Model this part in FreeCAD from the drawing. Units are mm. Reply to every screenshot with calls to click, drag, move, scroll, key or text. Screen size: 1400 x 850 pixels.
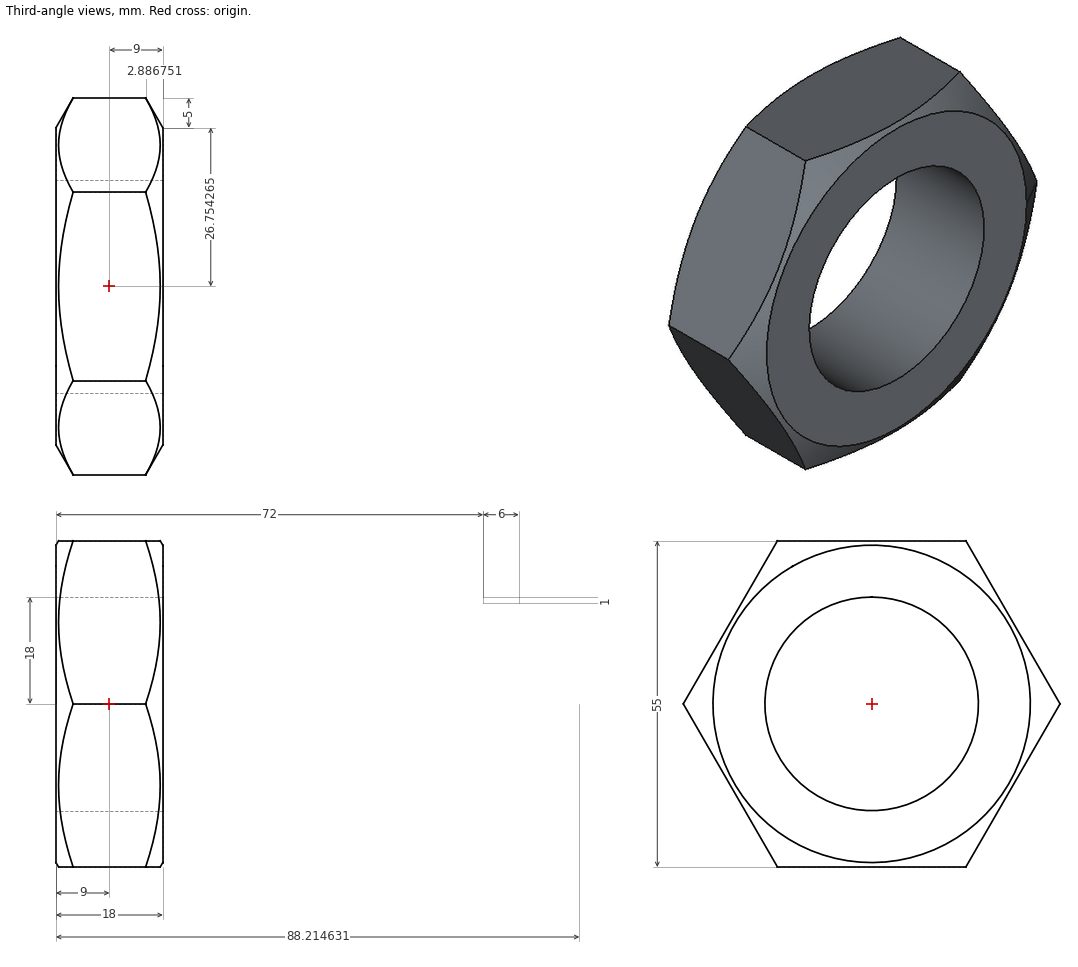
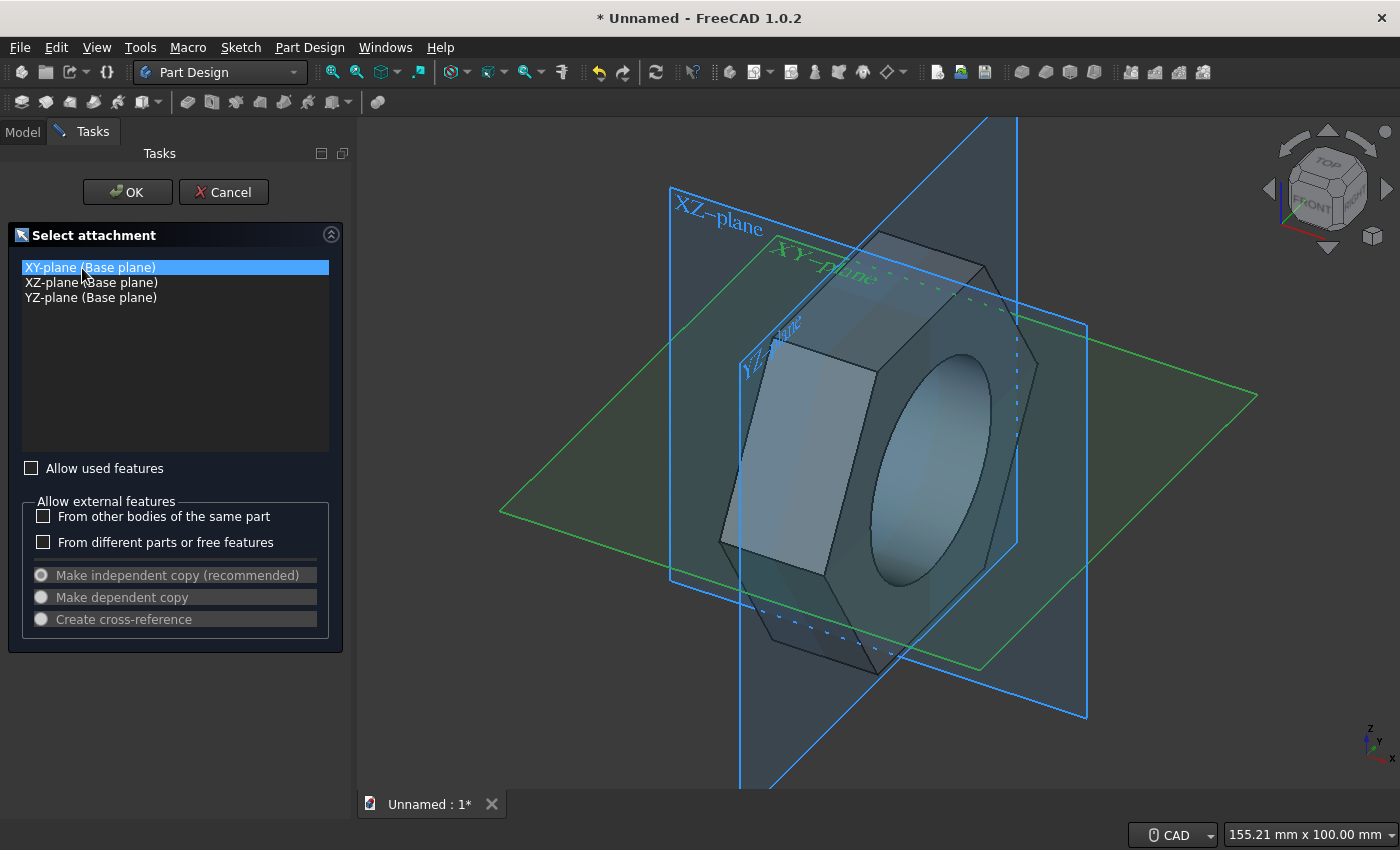
click(128, 192)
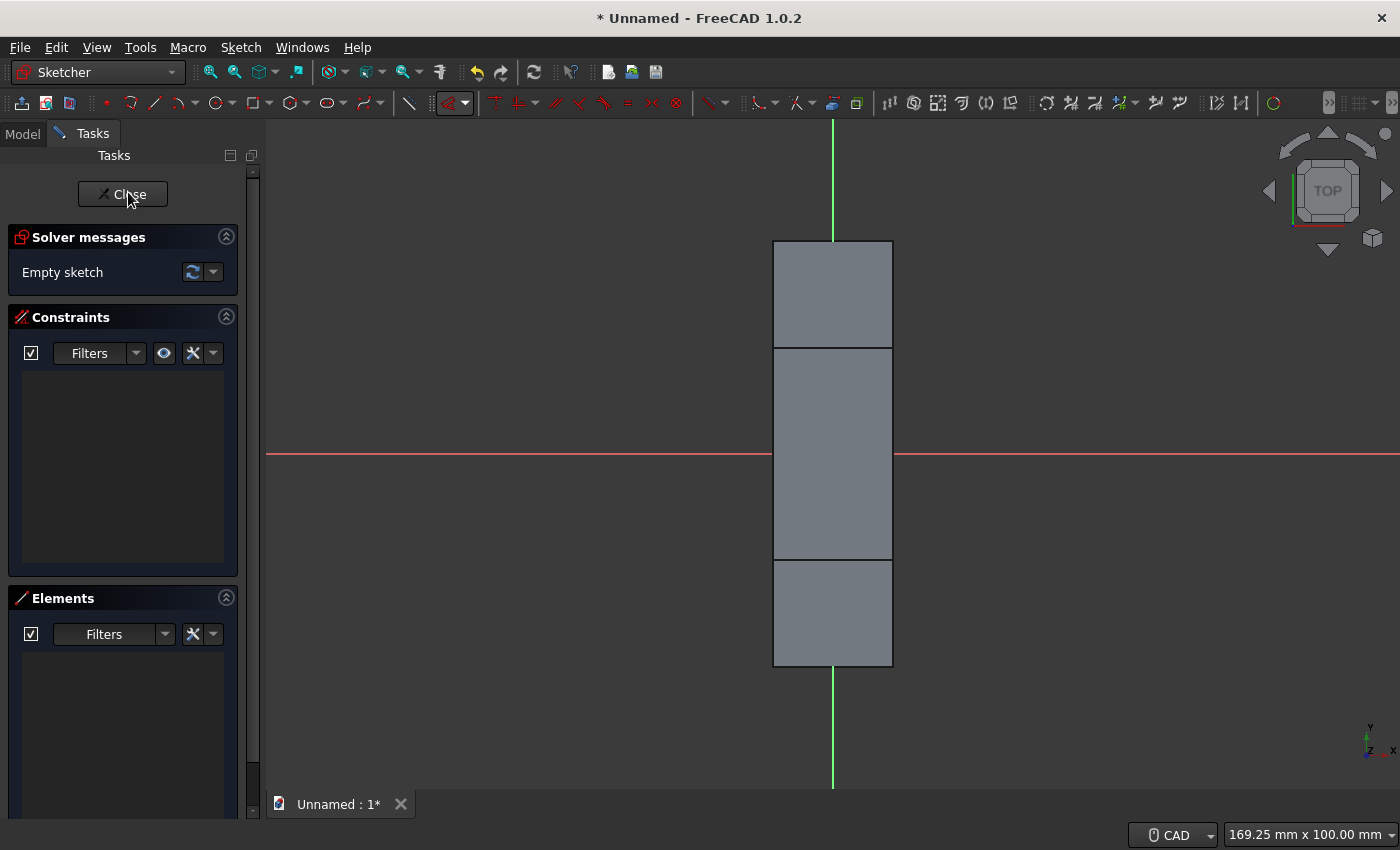
click(70, 104)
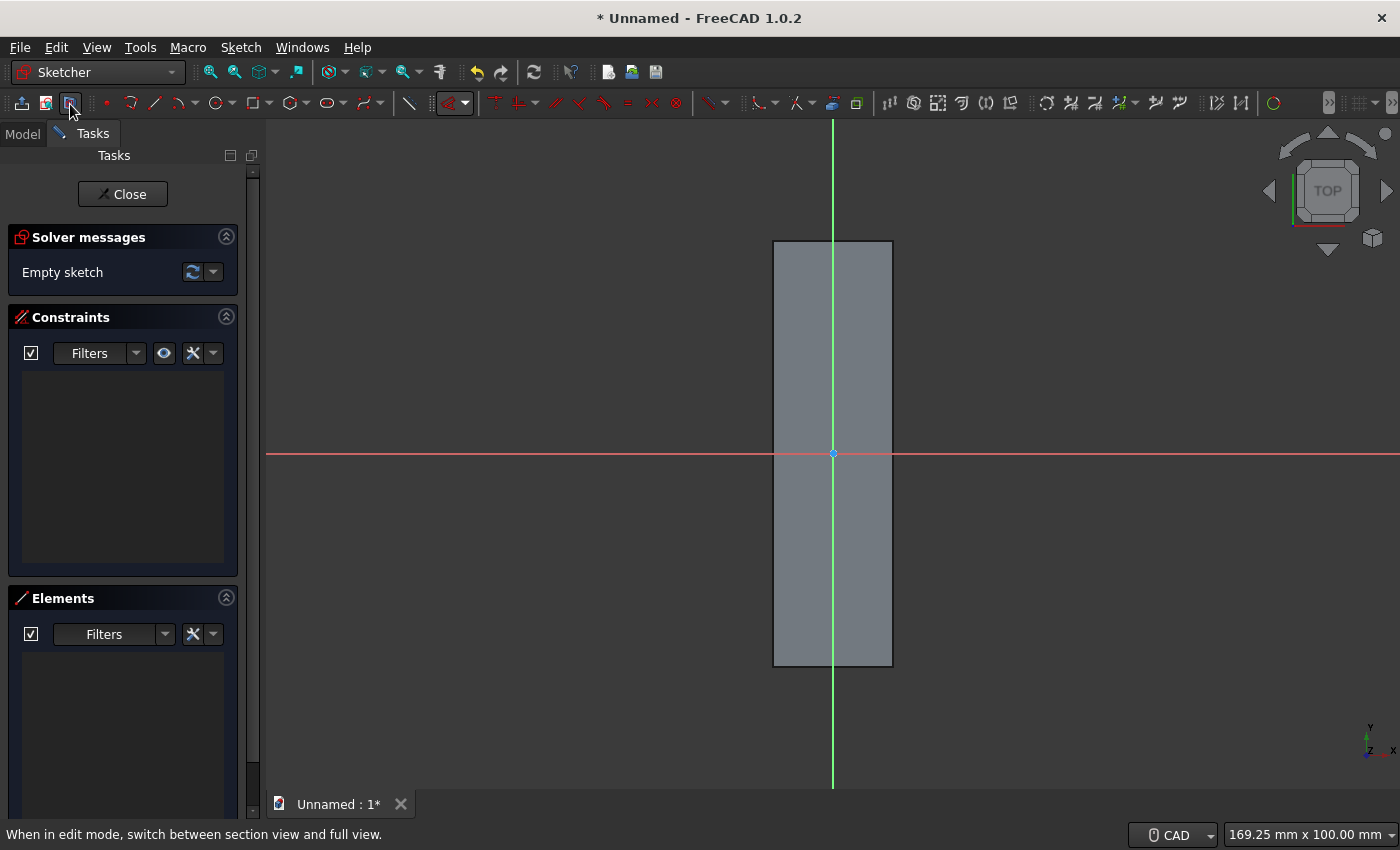
scroll(893, 242, up, 13)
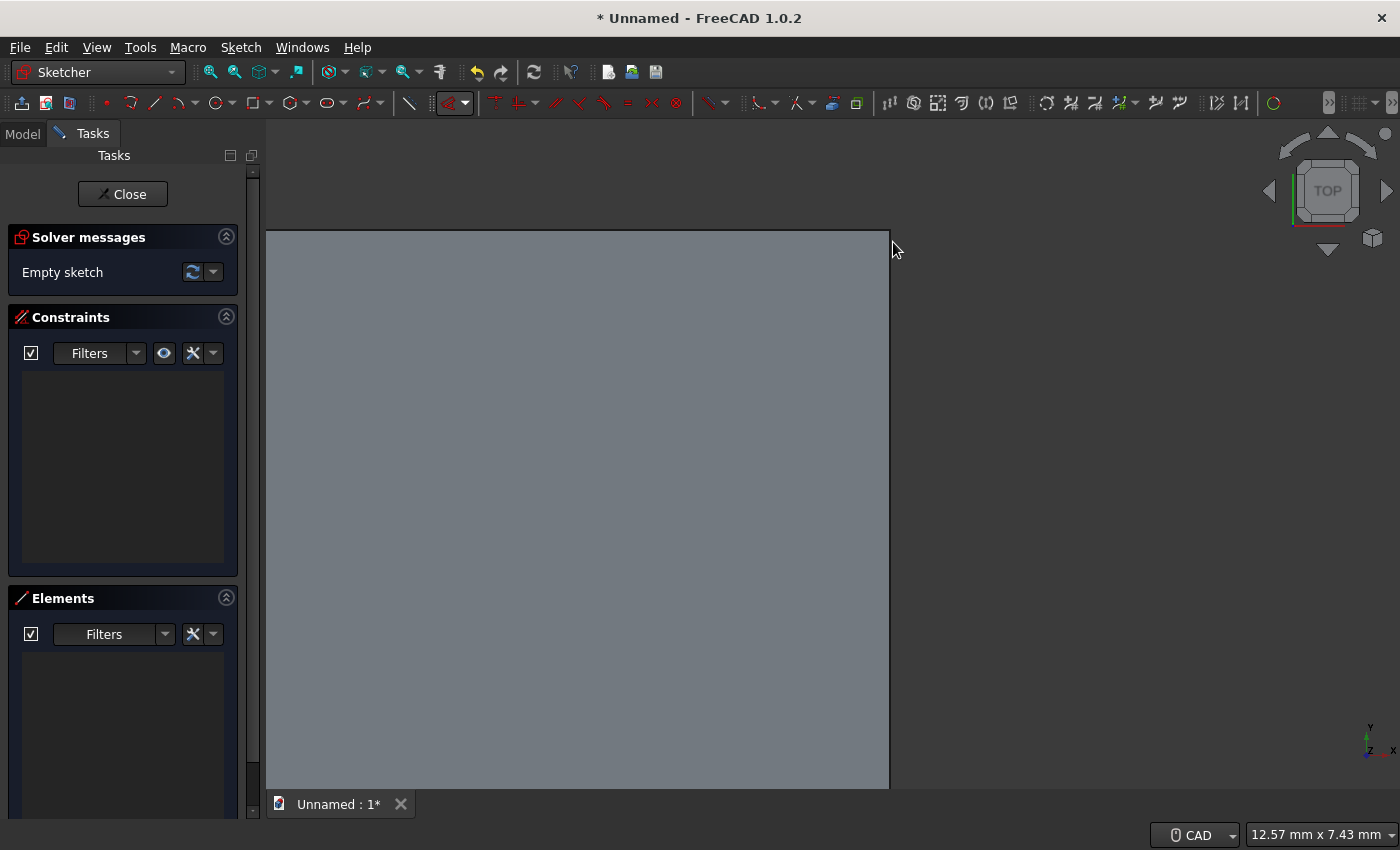
click(132, 104)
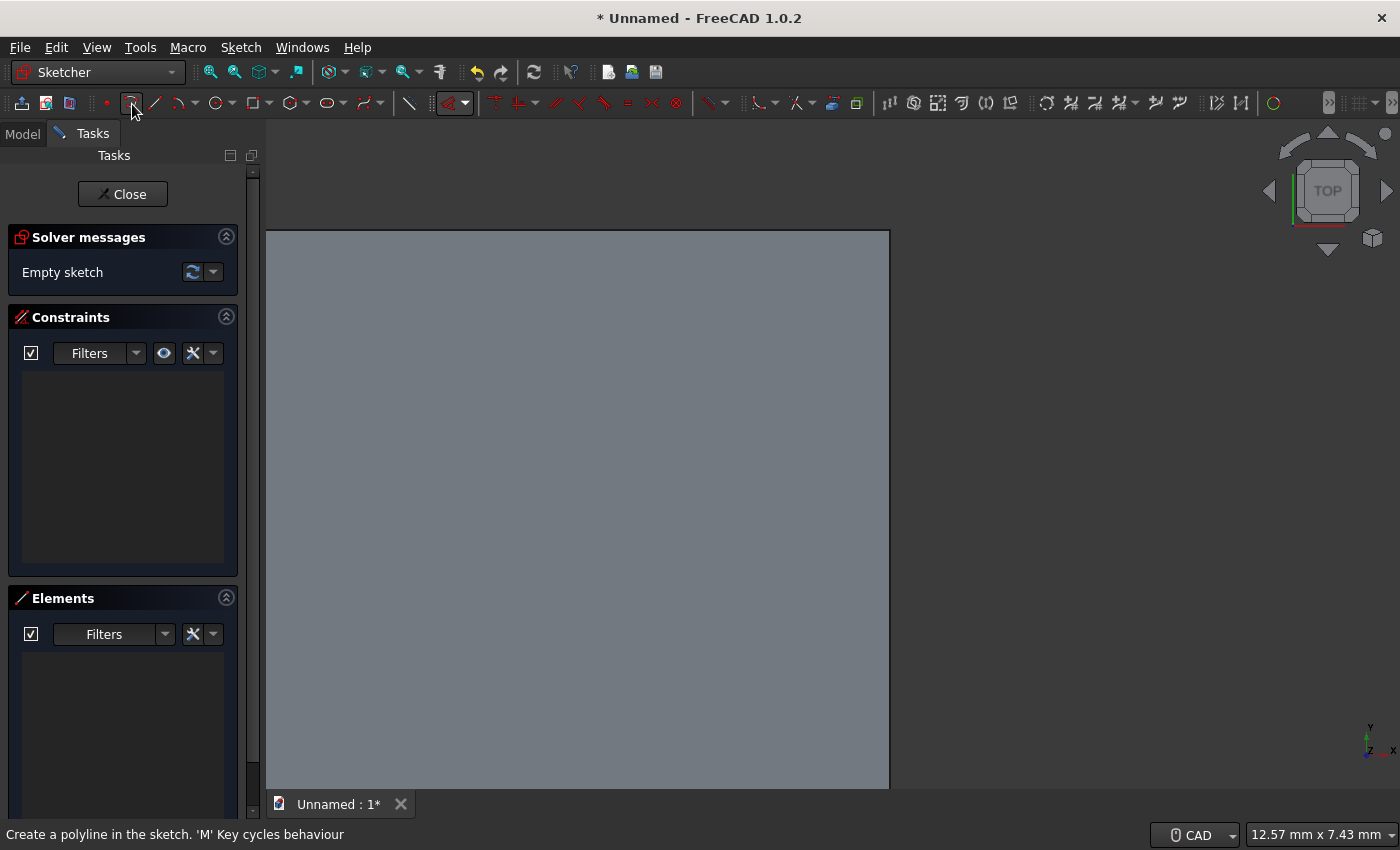
click(890, 681)
click(890, 230)
click(630, 230)
click(890, 682)
key(Escape)
key(Escape)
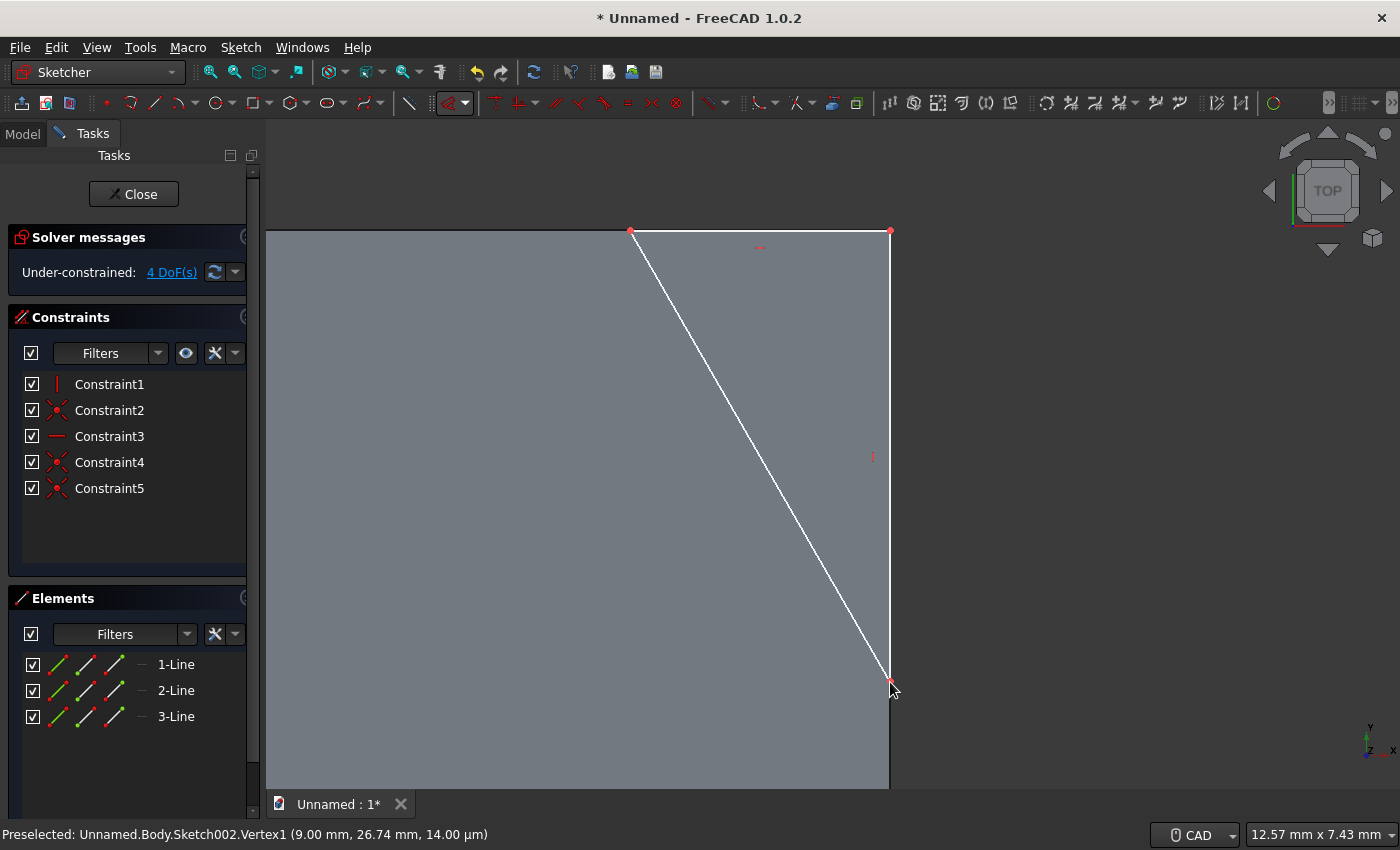
click(890, 547)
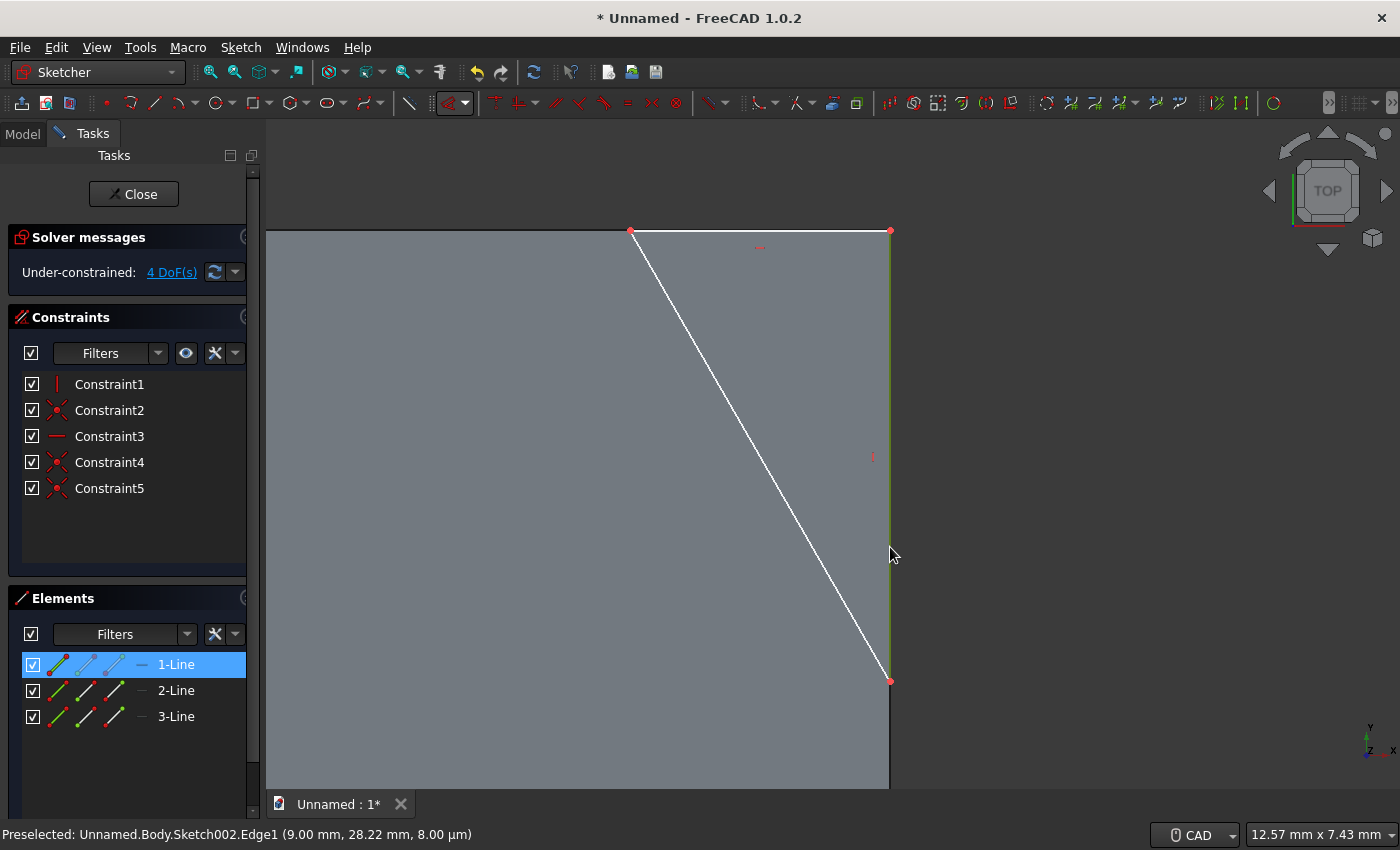
key(i)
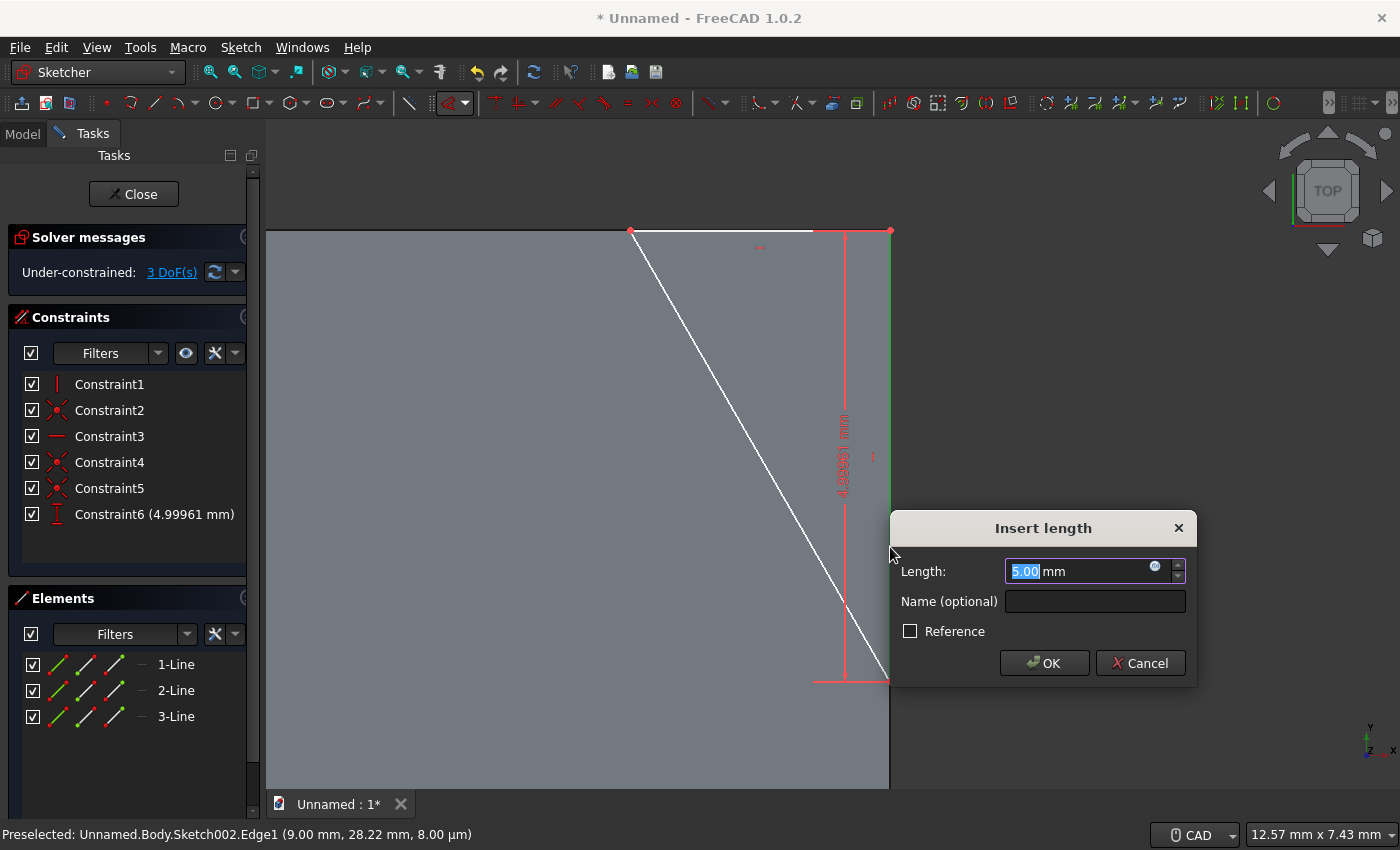
text(5)
key(Return)